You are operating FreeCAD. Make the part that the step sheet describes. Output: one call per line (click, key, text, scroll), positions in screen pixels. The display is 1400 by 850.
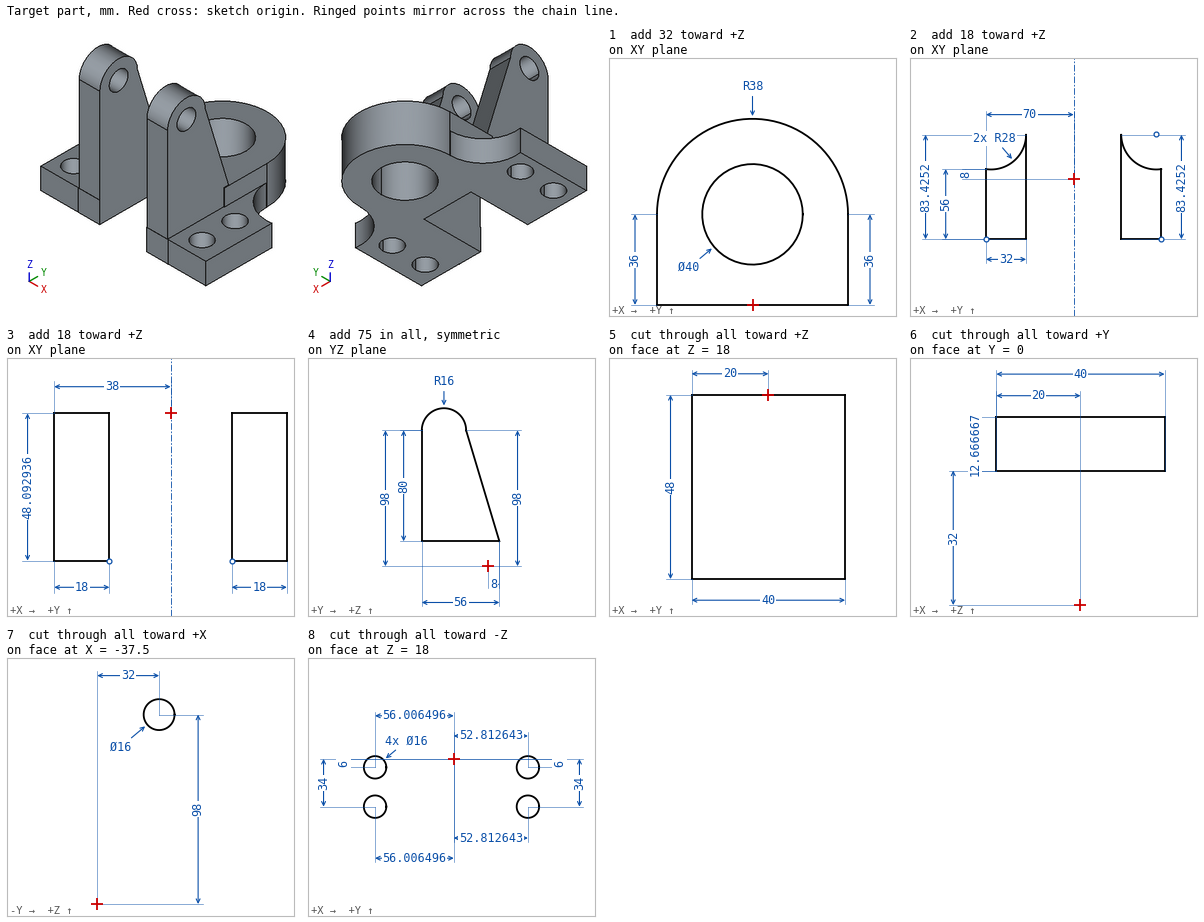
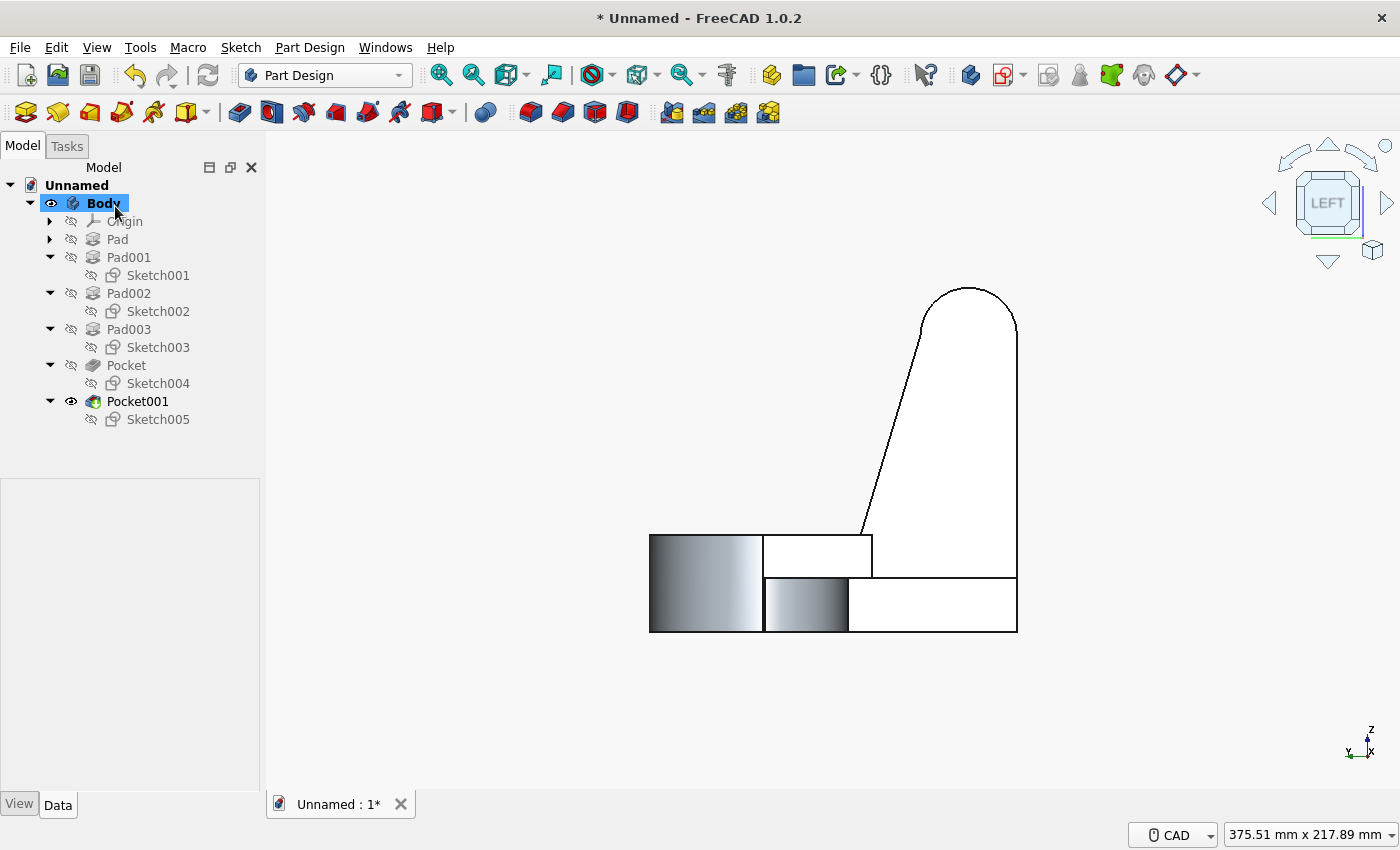
click(939, 514)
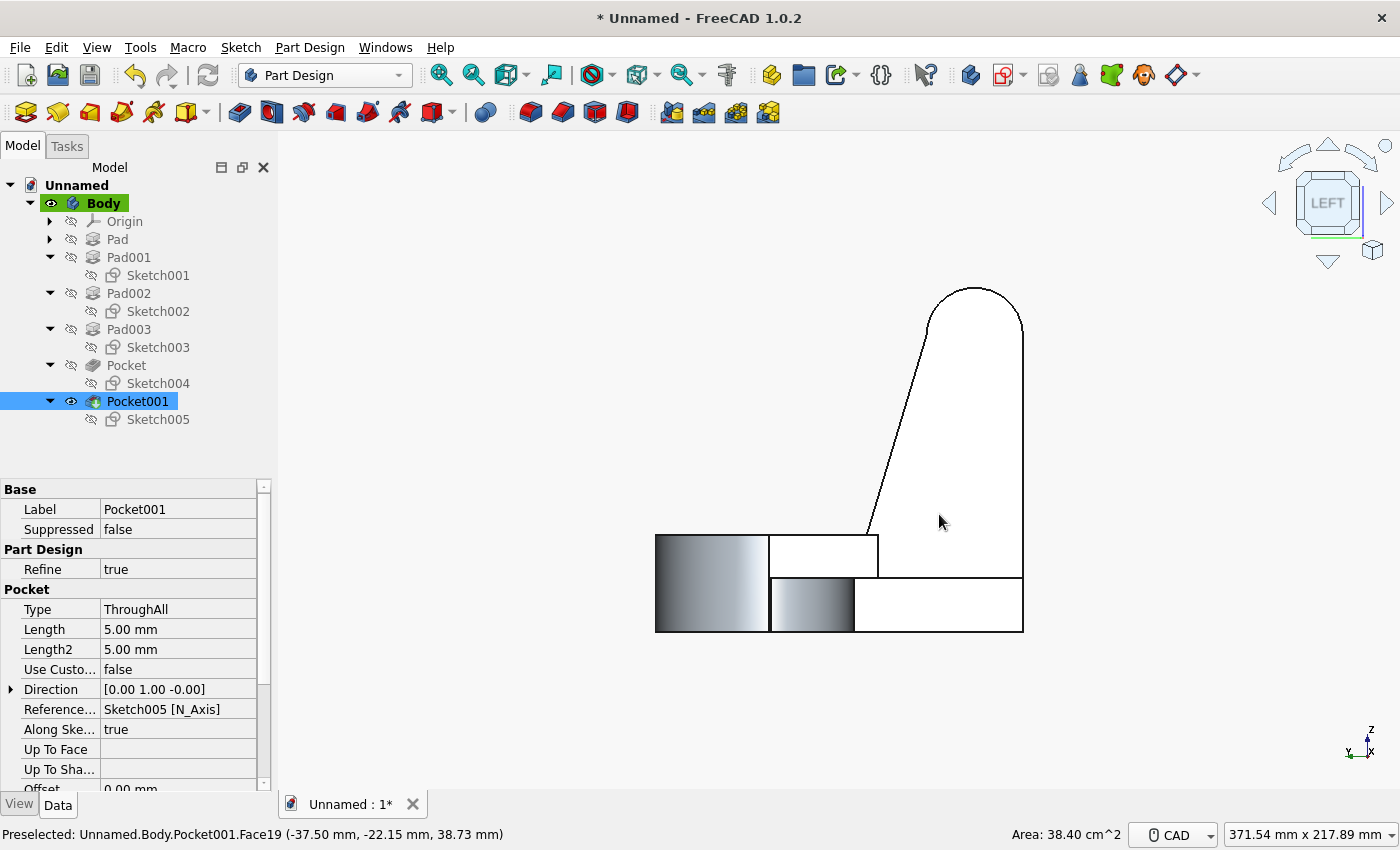
click(1004, 76)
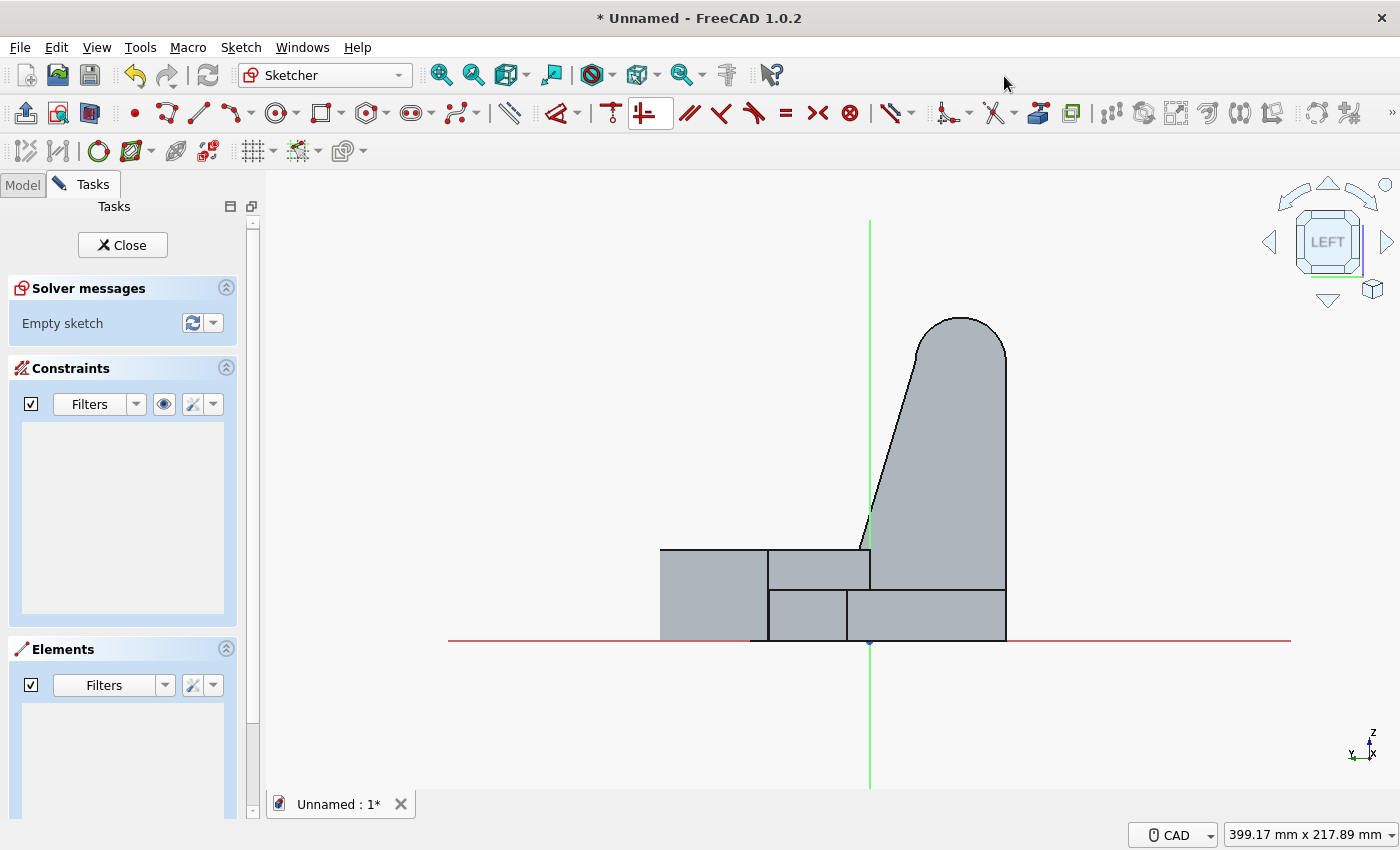
scroll(985, 348, up, 11)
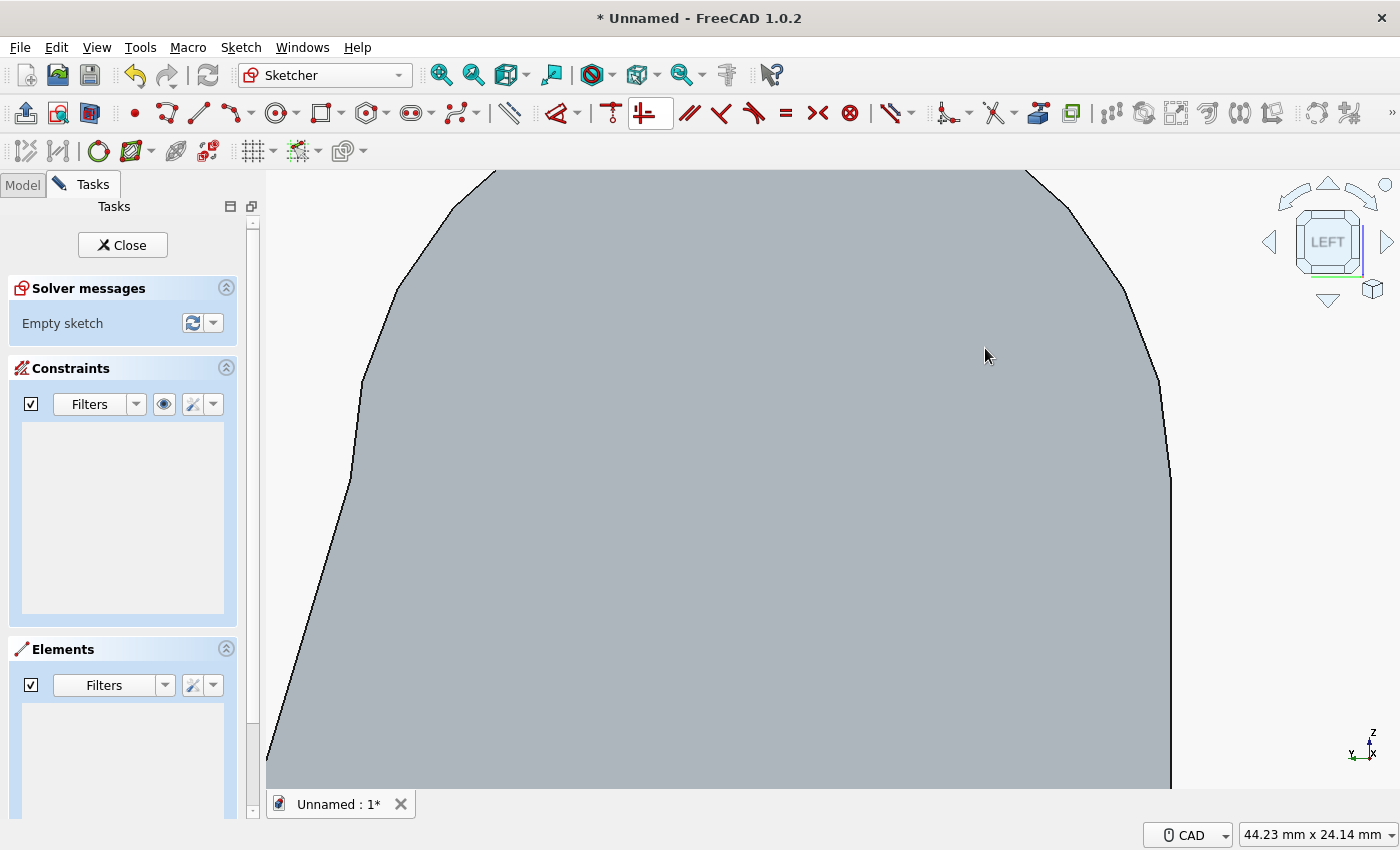
click(276, 114)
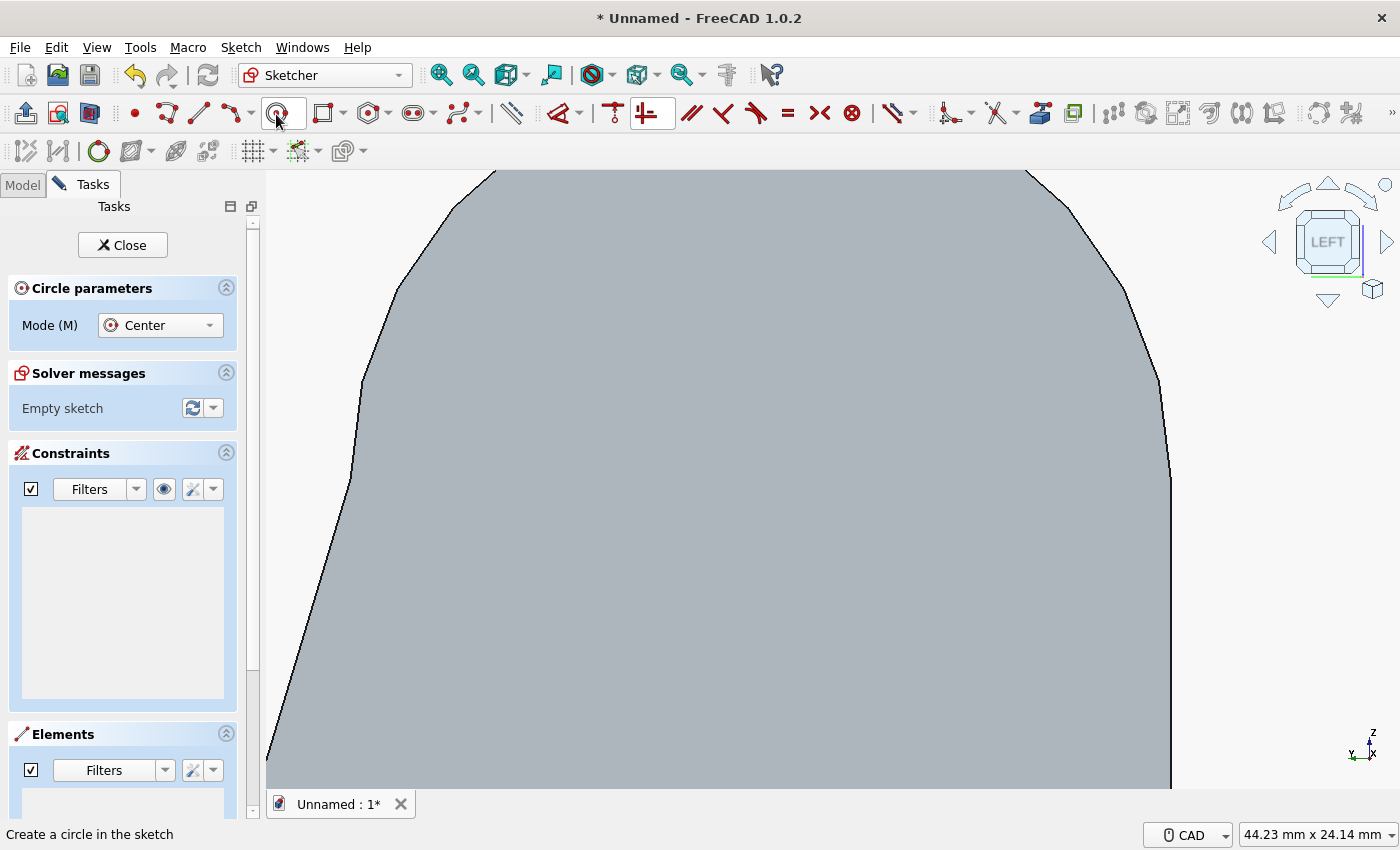
click(761, 480)
click(906, 335)
key(Escape)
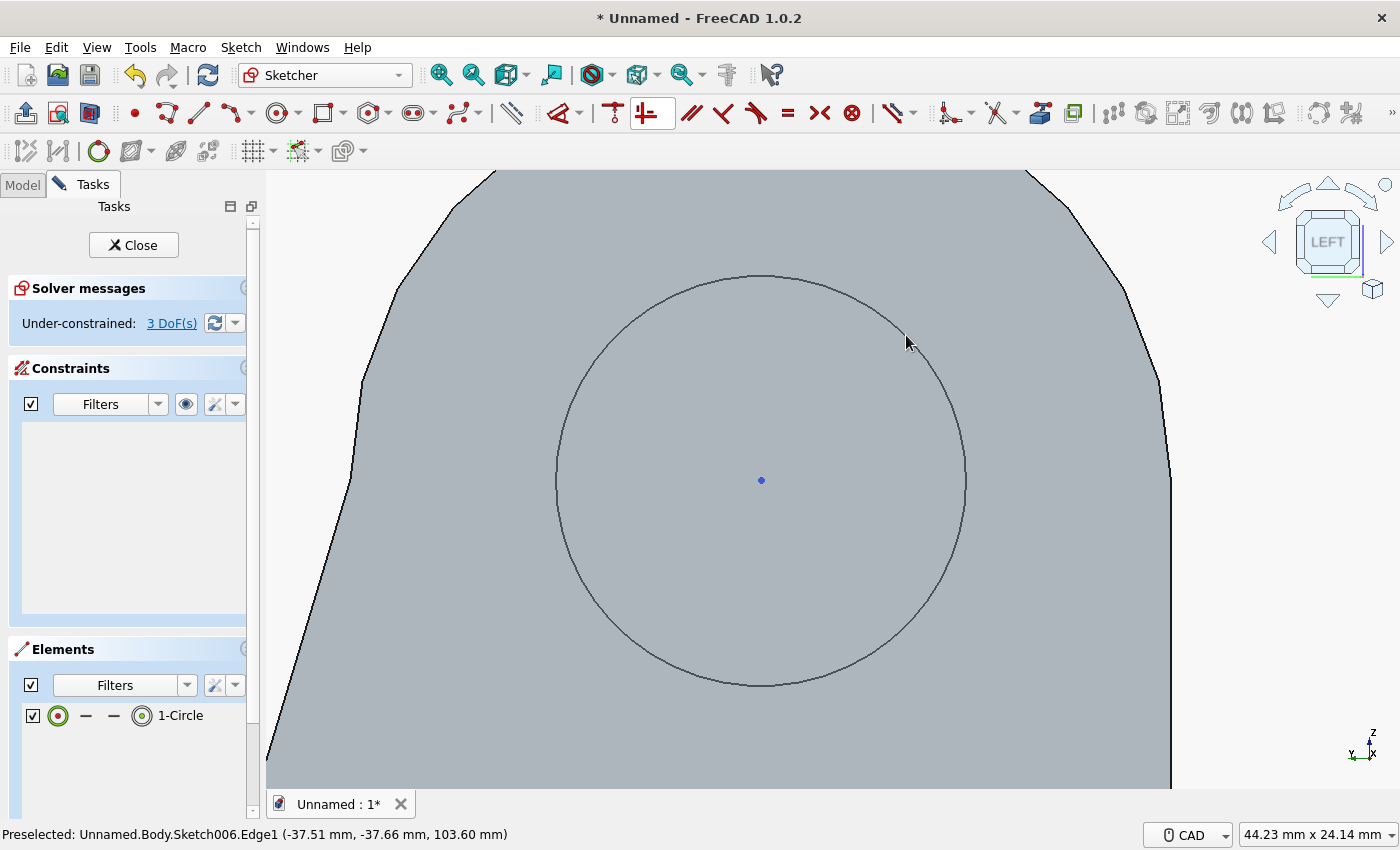
click(558, 114)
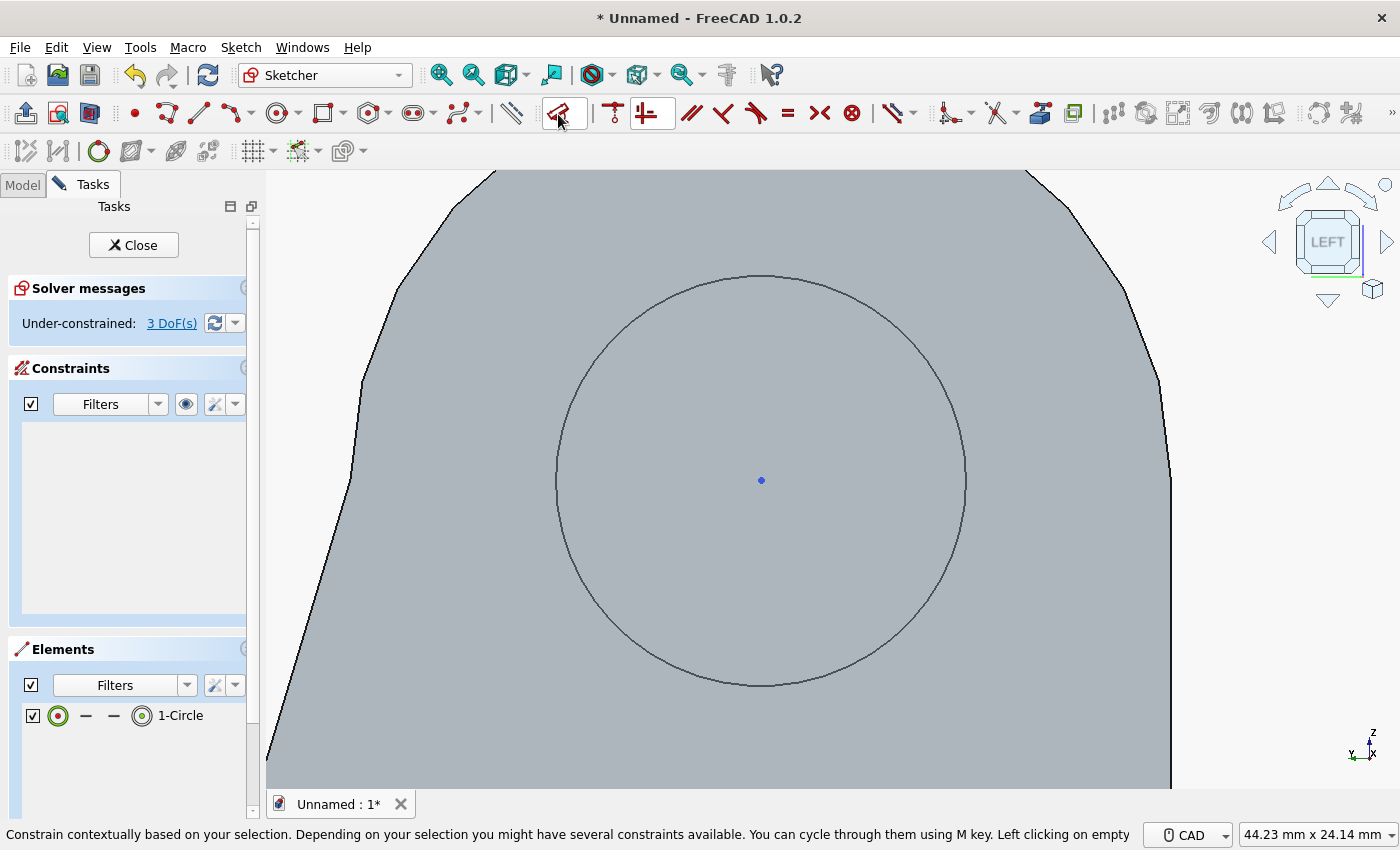
click(906, 336)
click(929, 313)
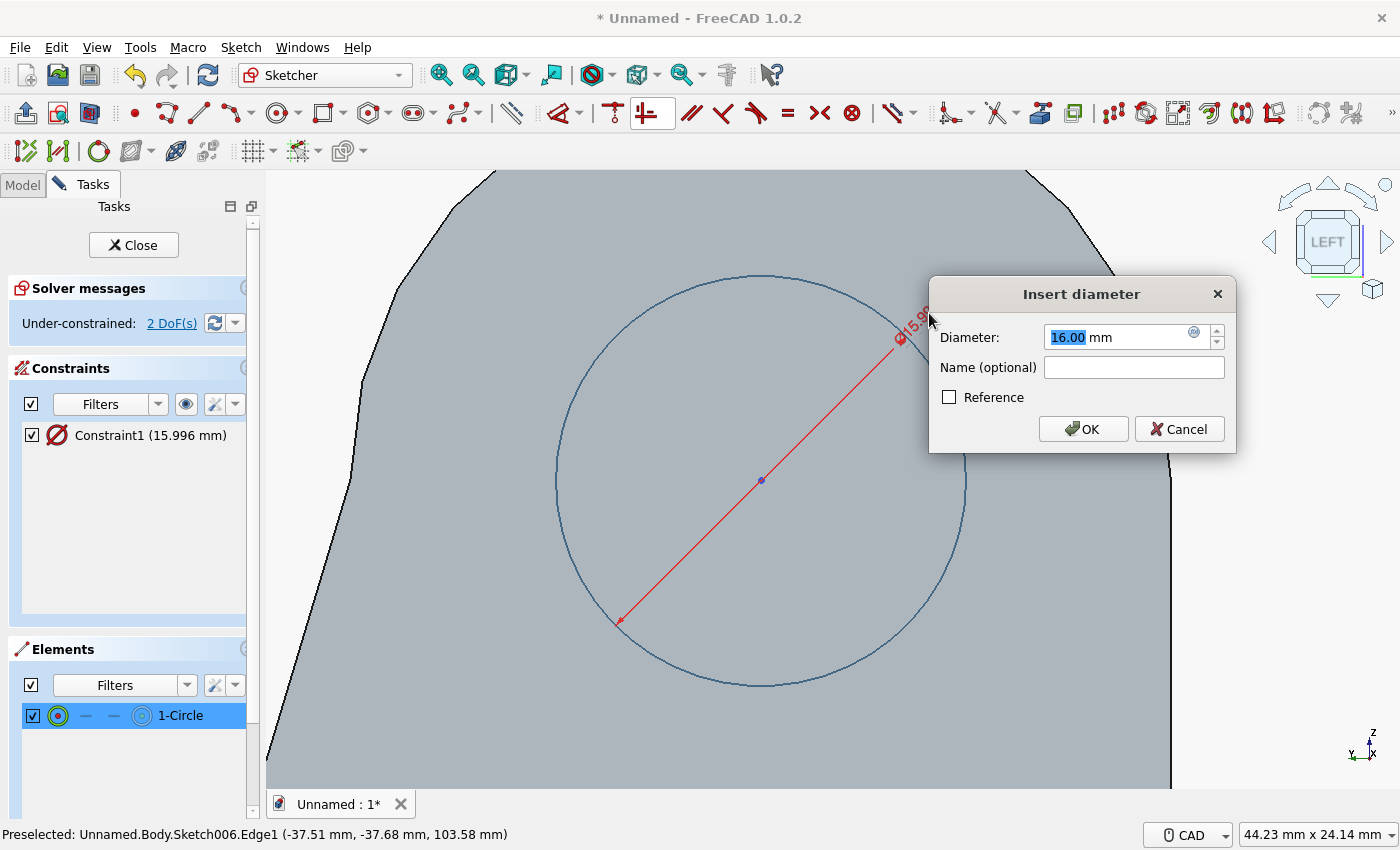
text(16)
key(Return)